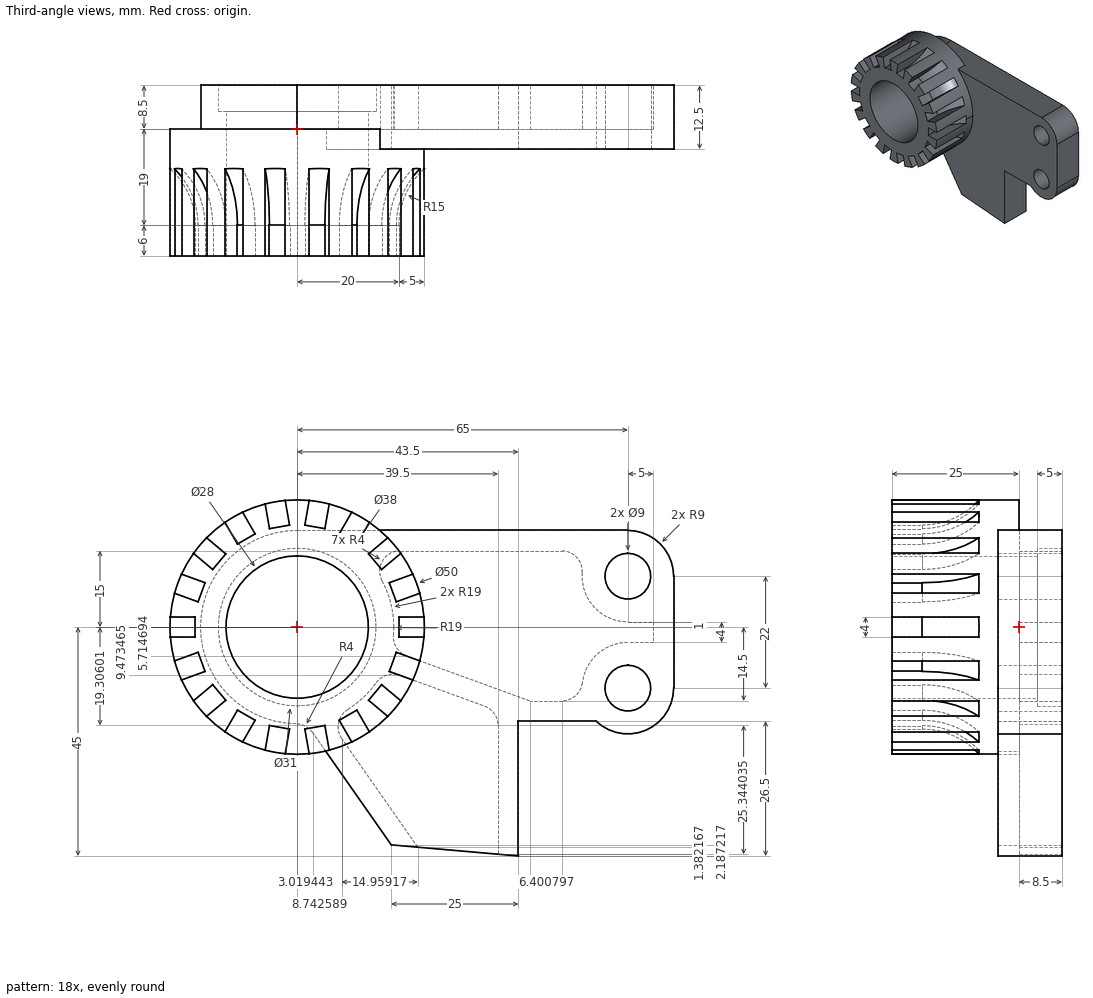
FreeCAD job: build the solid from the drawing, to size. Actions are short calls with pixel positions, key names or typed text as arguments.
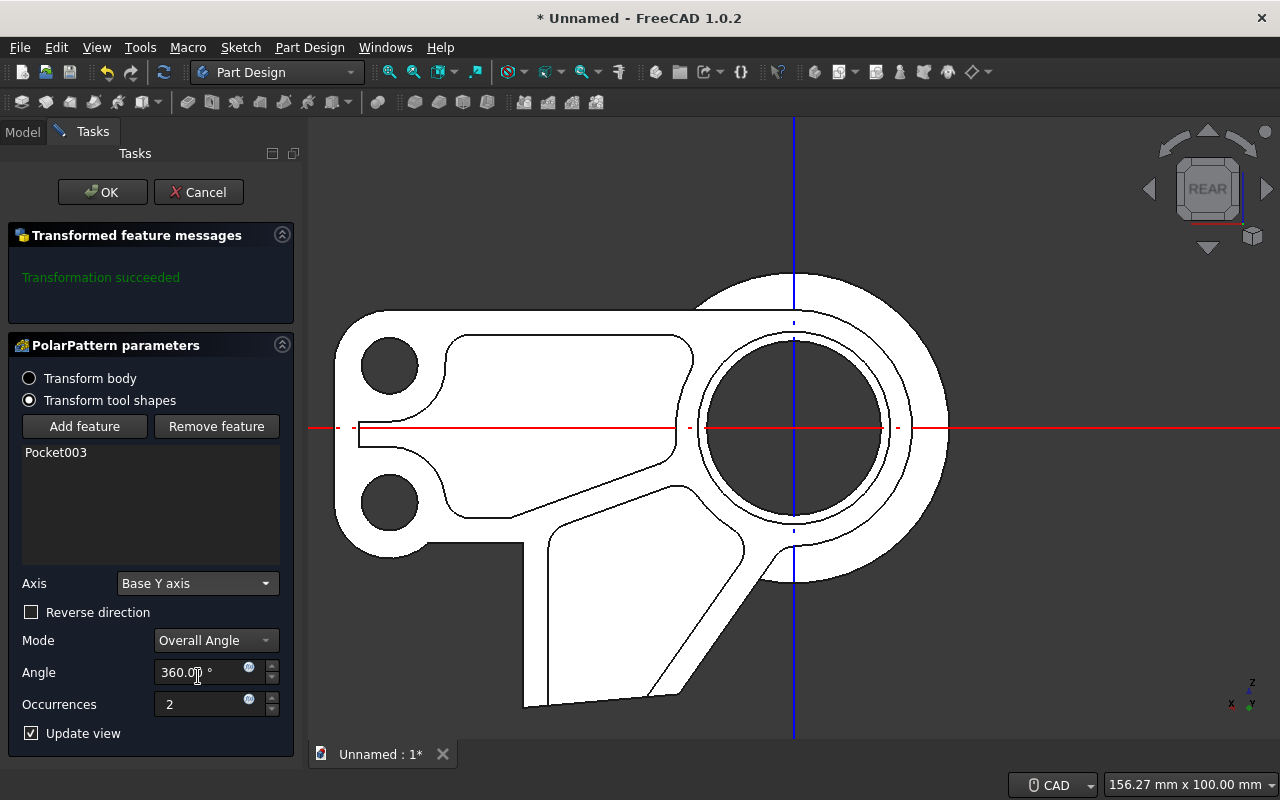
triple_click(209, 704)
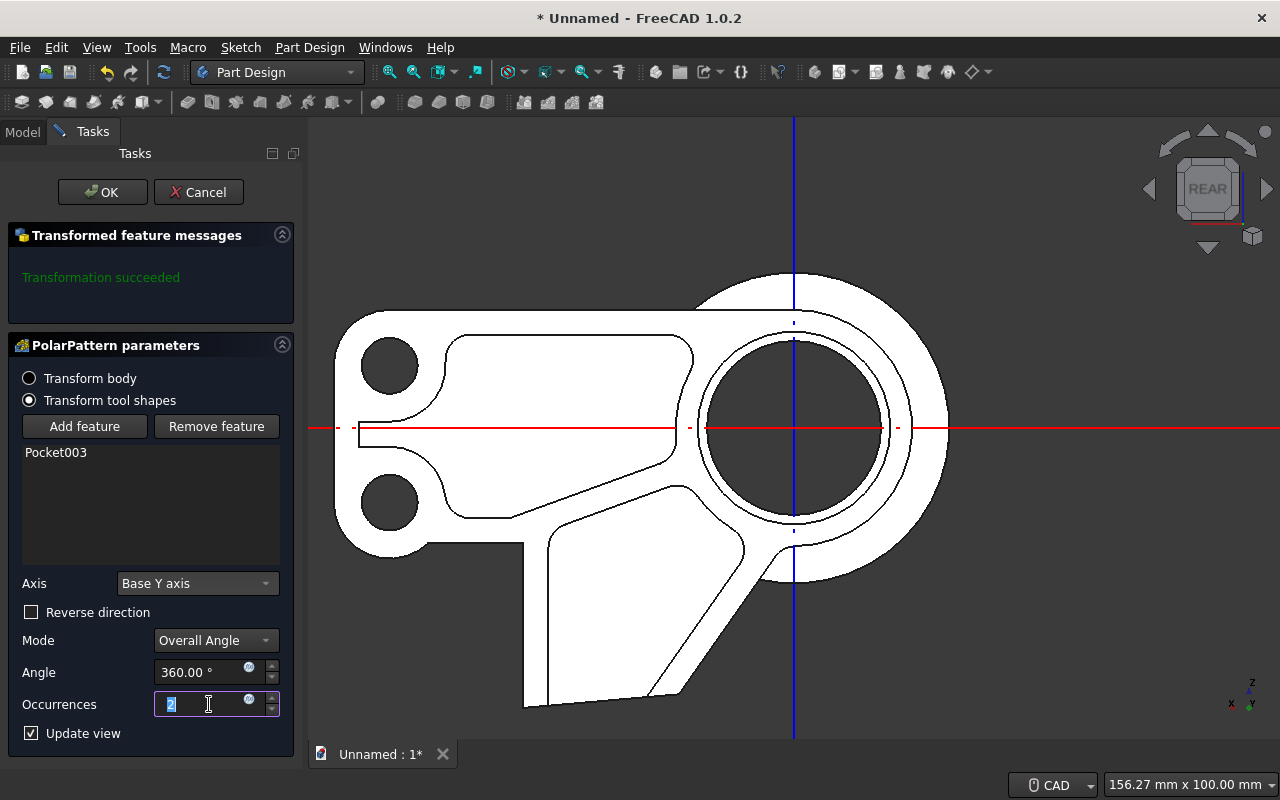
text(18)
key(Tab)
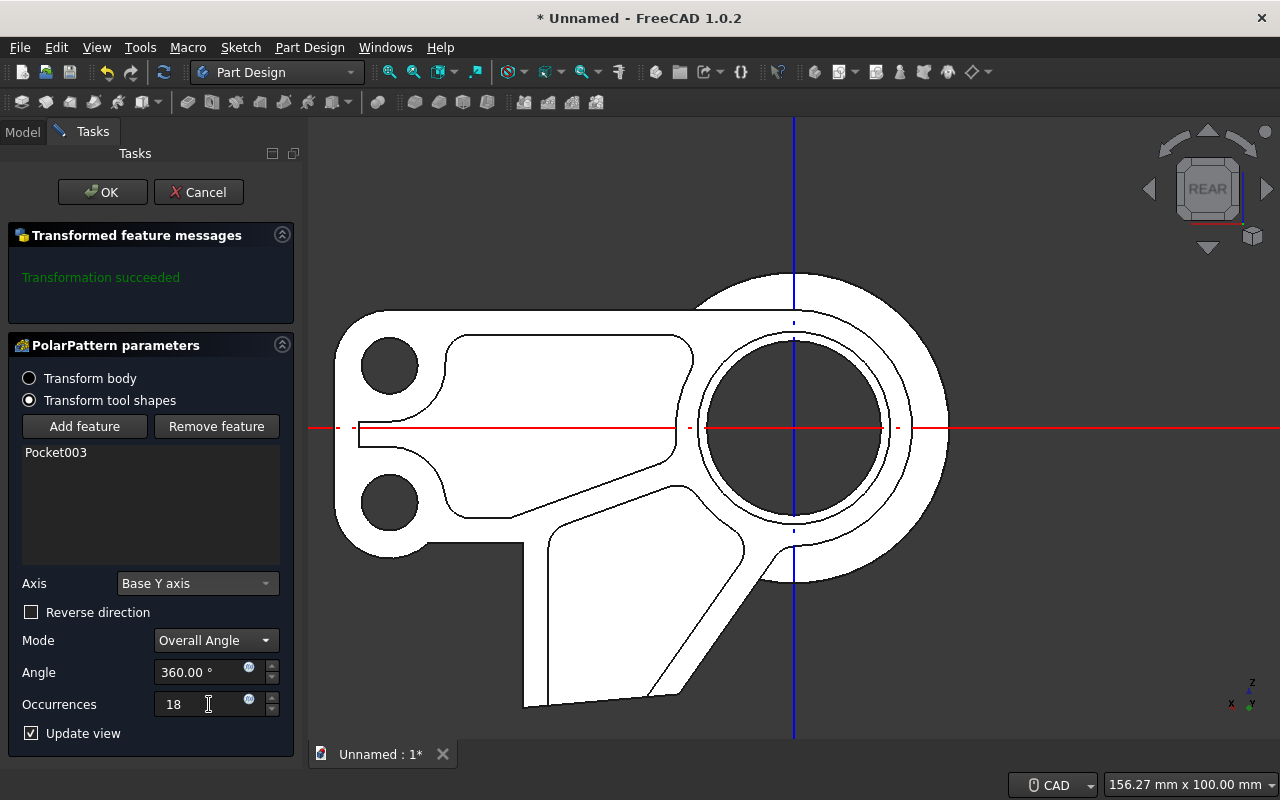
click(103, 192)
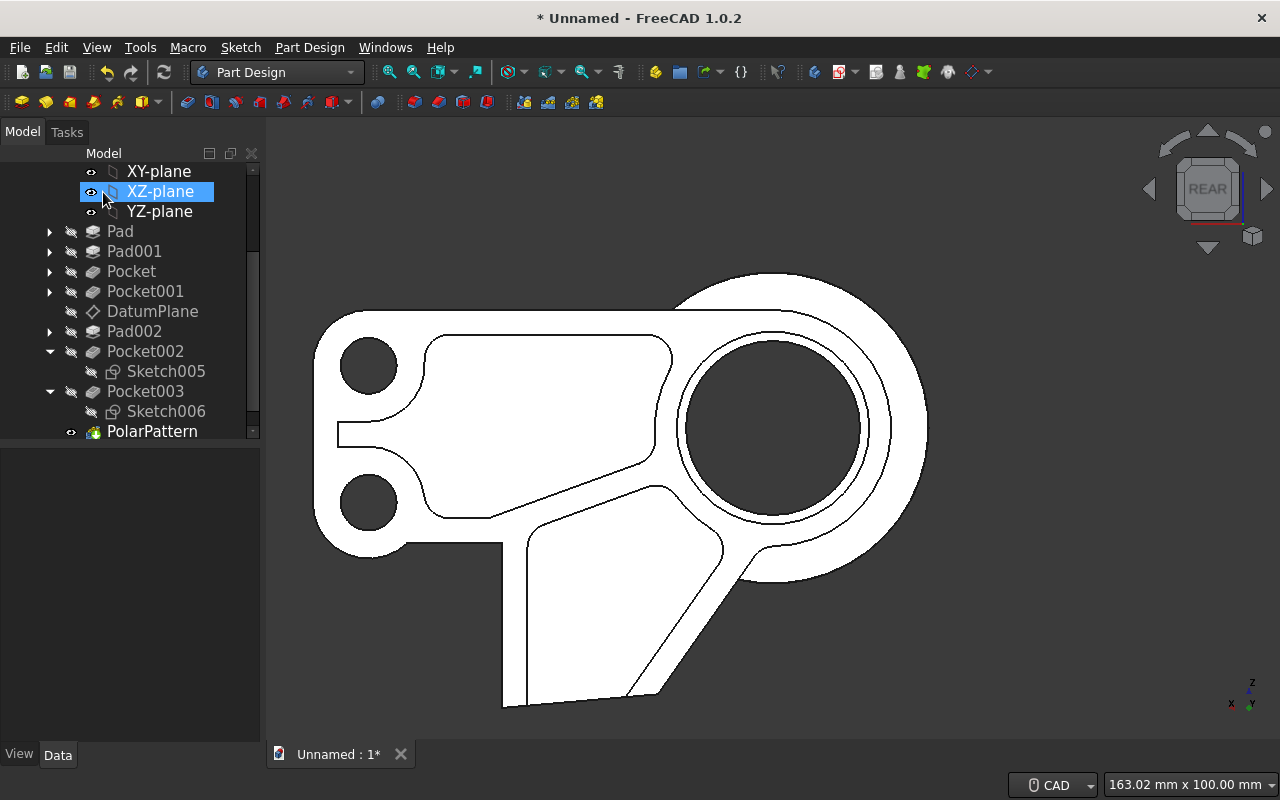
key(0)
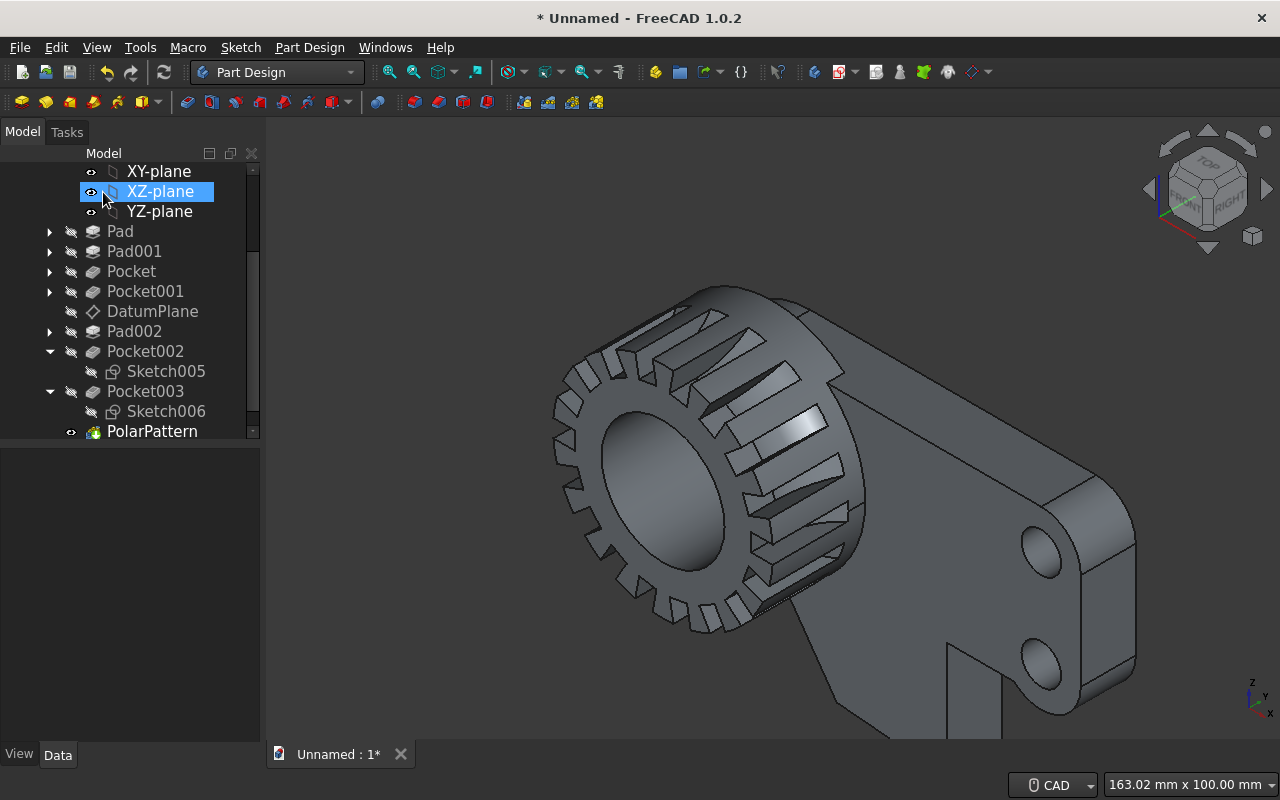
click(390, 72)